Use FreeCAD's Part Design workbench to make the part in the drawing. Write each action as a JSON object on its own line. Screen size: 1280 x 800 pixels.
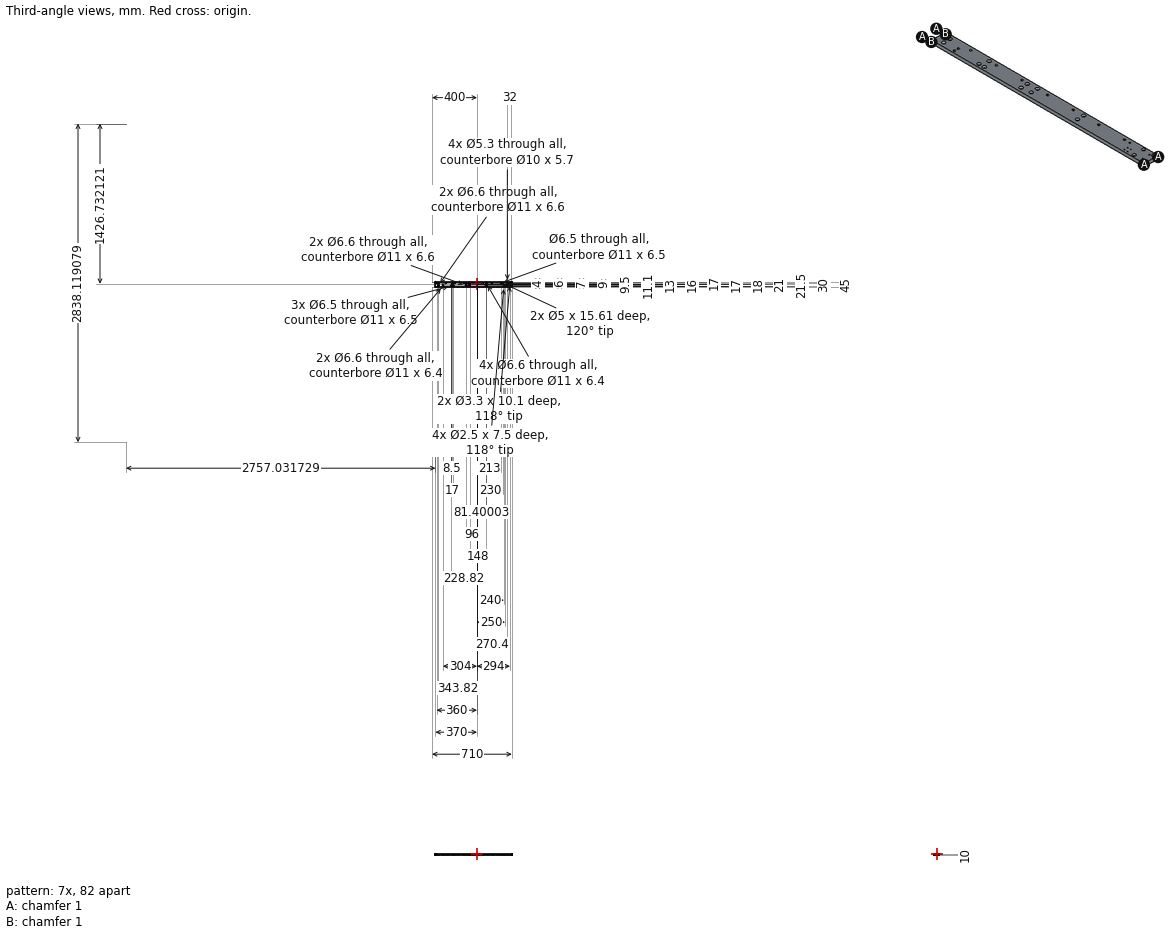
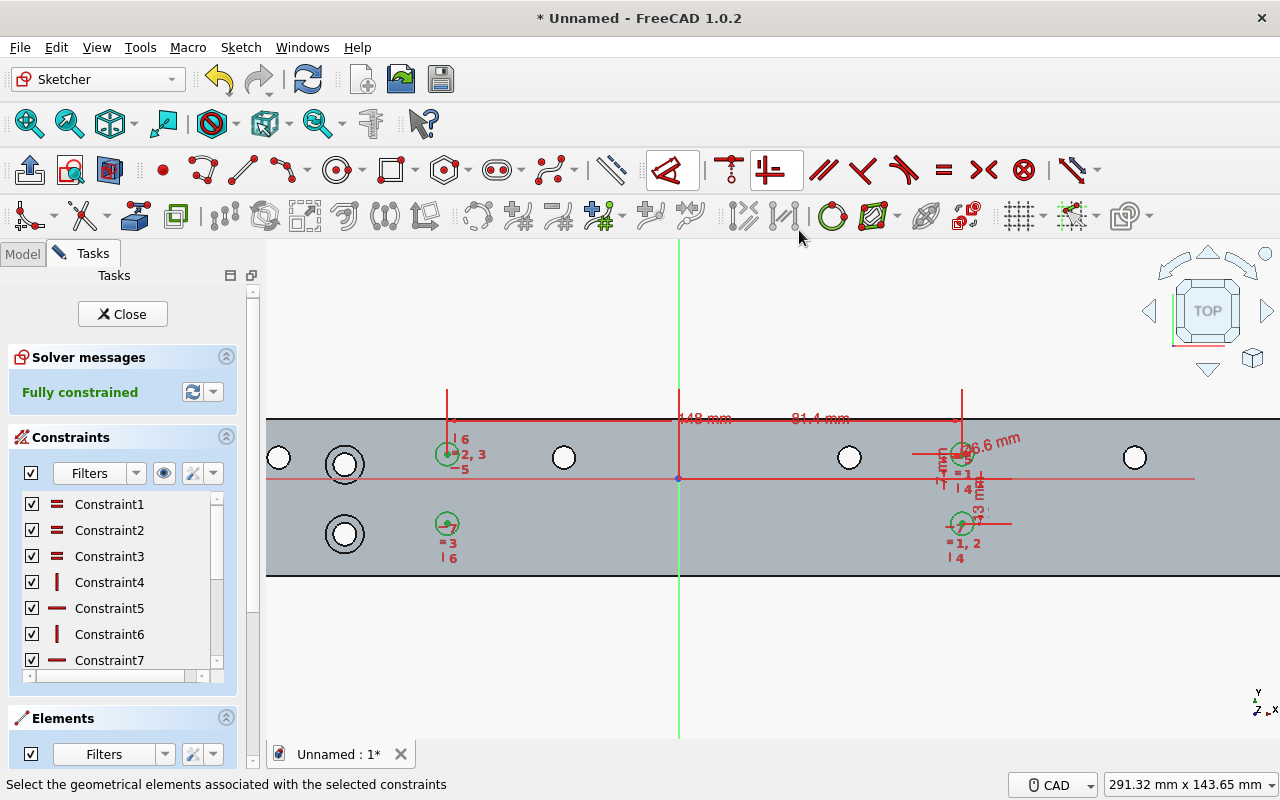
{"action": "left_click", "coordinate": [123, 314]}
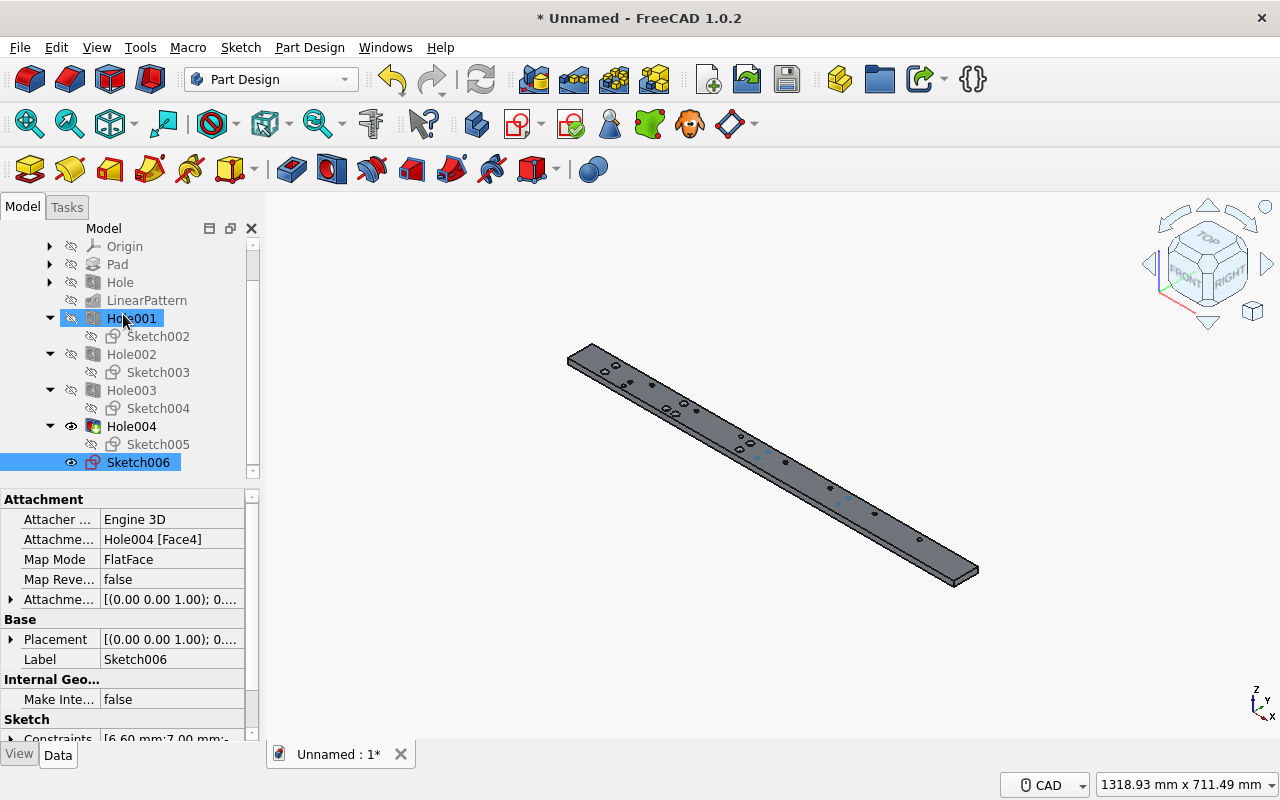
{"action": "left_click", "coordinate": [332, 170]}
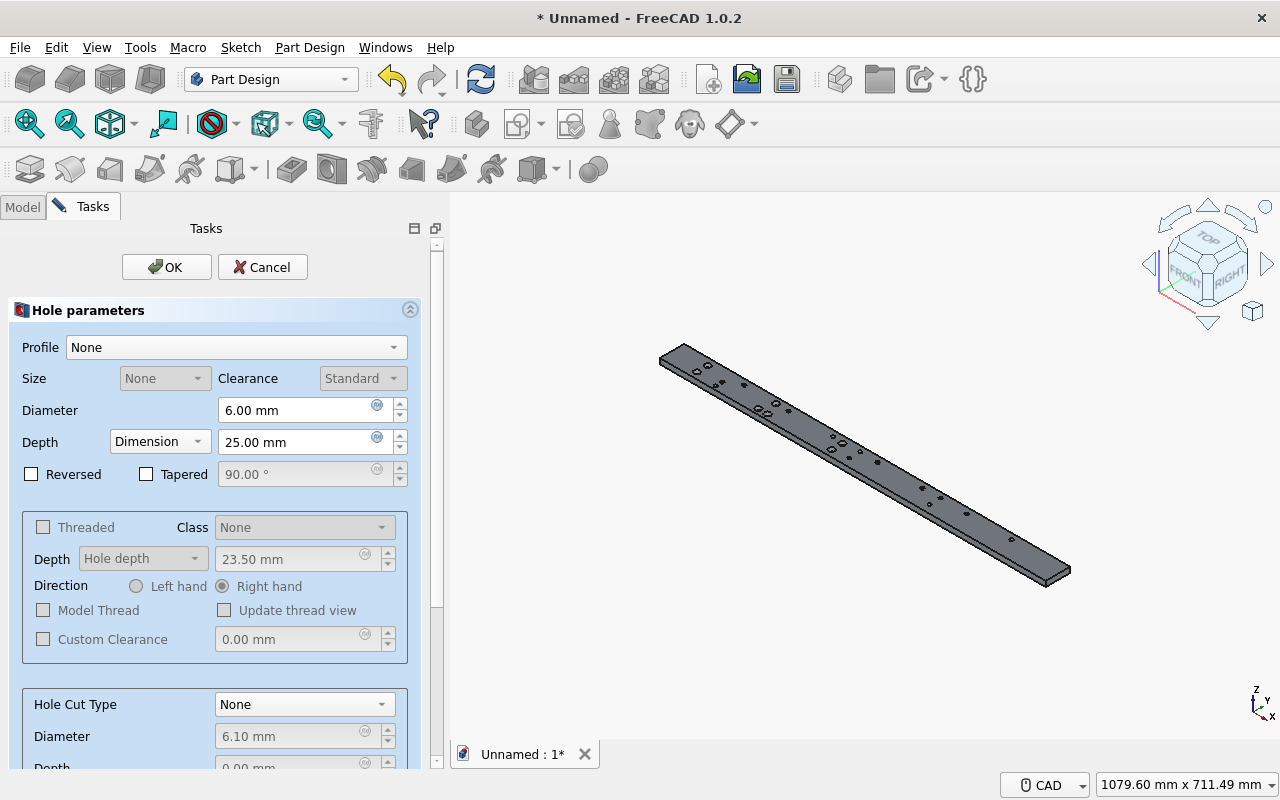
{"action": "triple_click", "coordinate": [305, 410]}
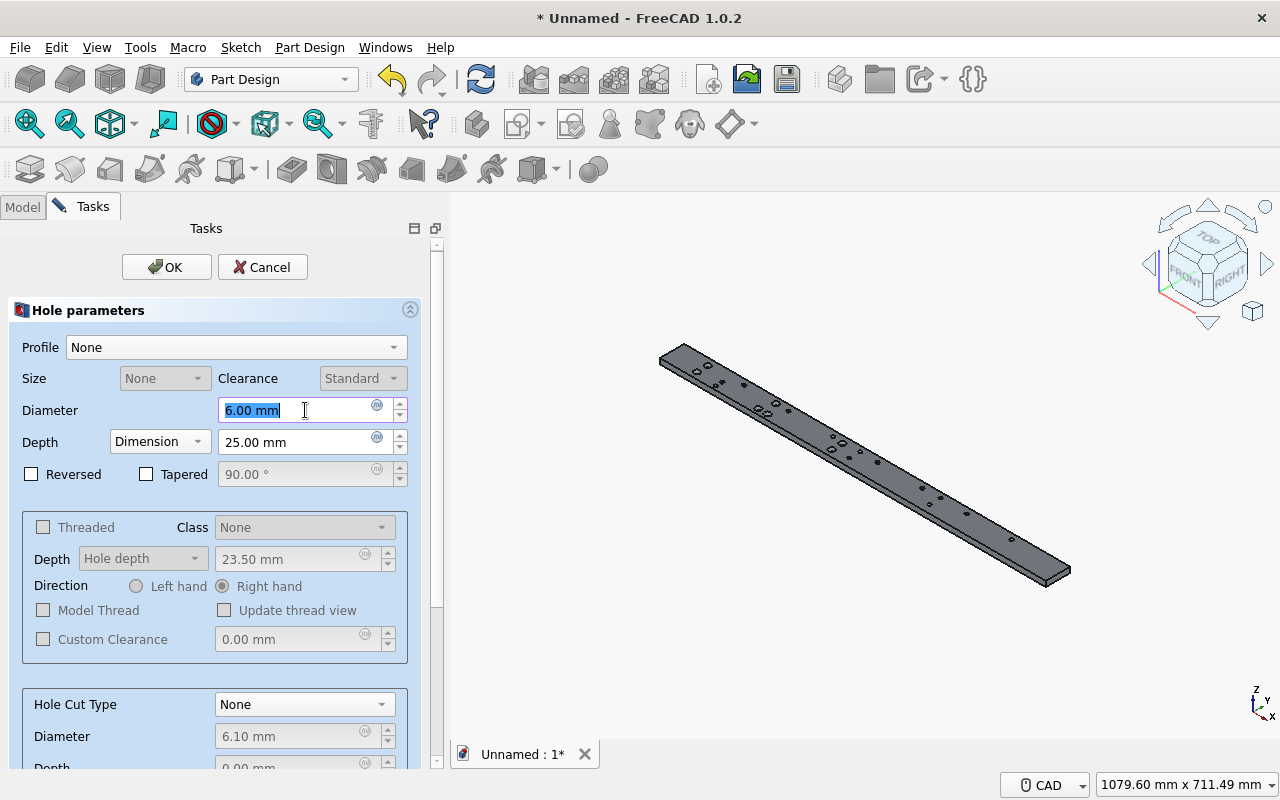
{"action": "type", "text": "6.6"}
{"action": "key", "text": "Tab"}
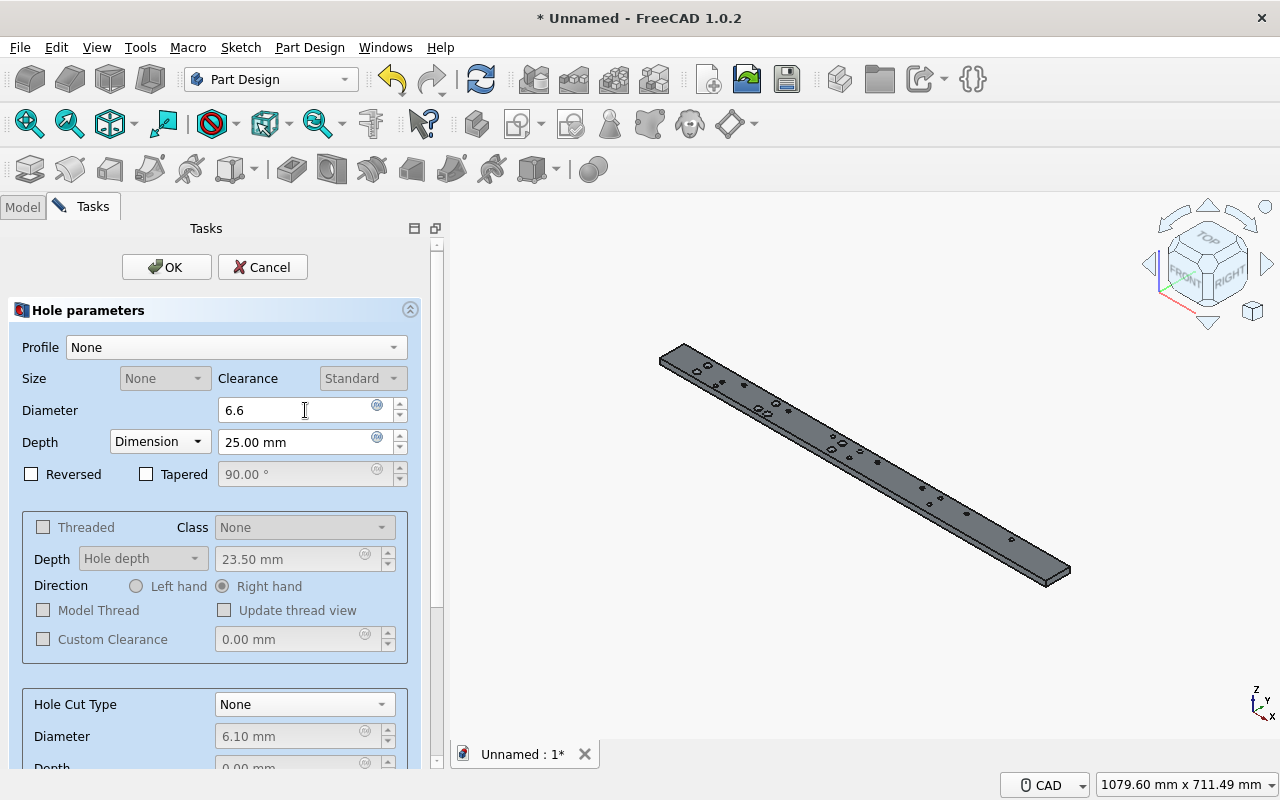
{"action": "left_click", "coordinate": [161, 442]}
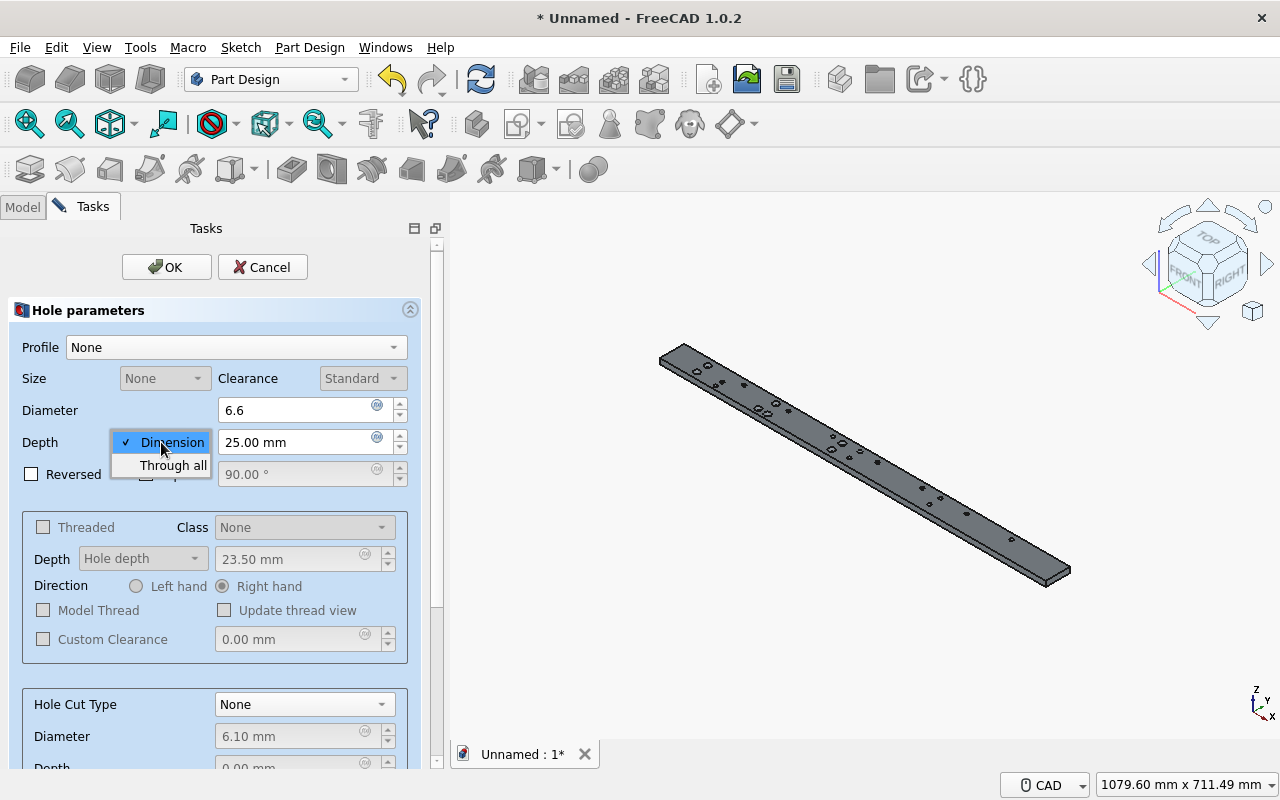
{"action": "left_click", "coordinate": [160, 466]}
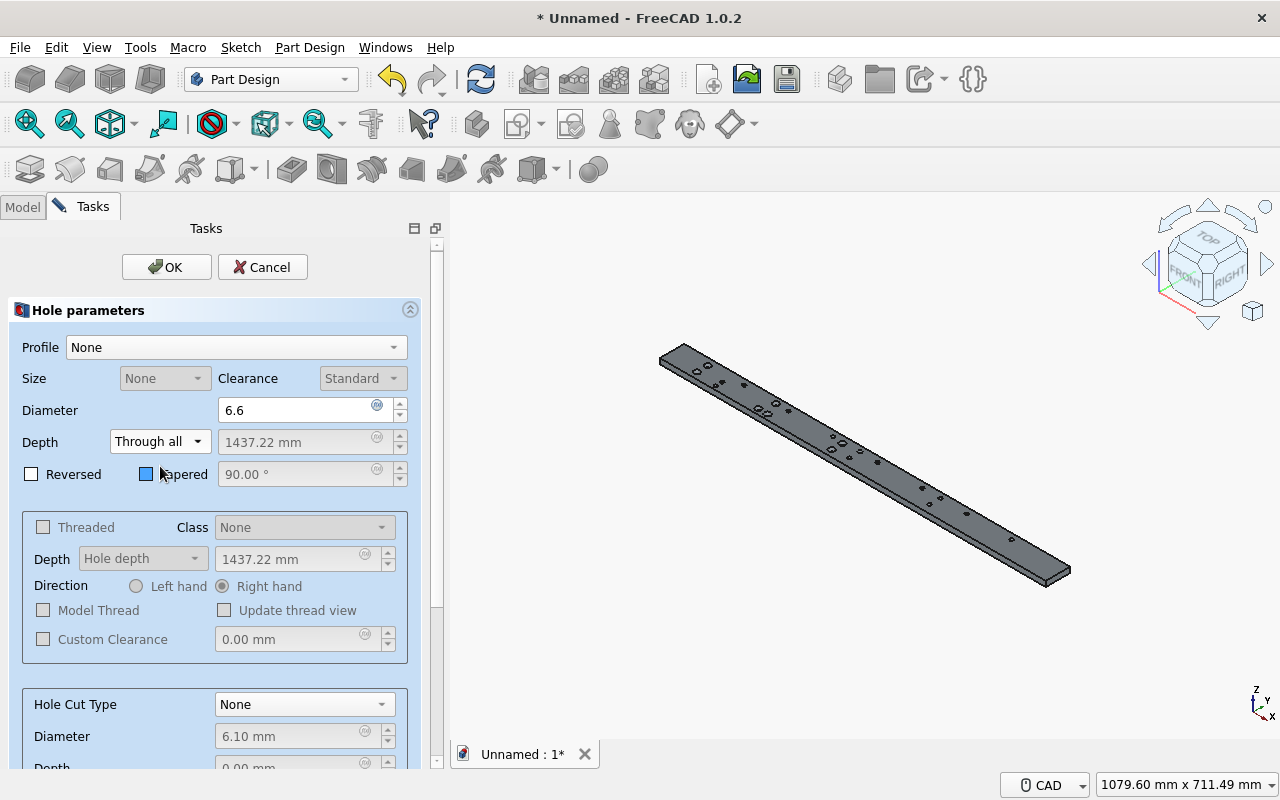
{"action": "left_click", "coordinate": [306, 704]}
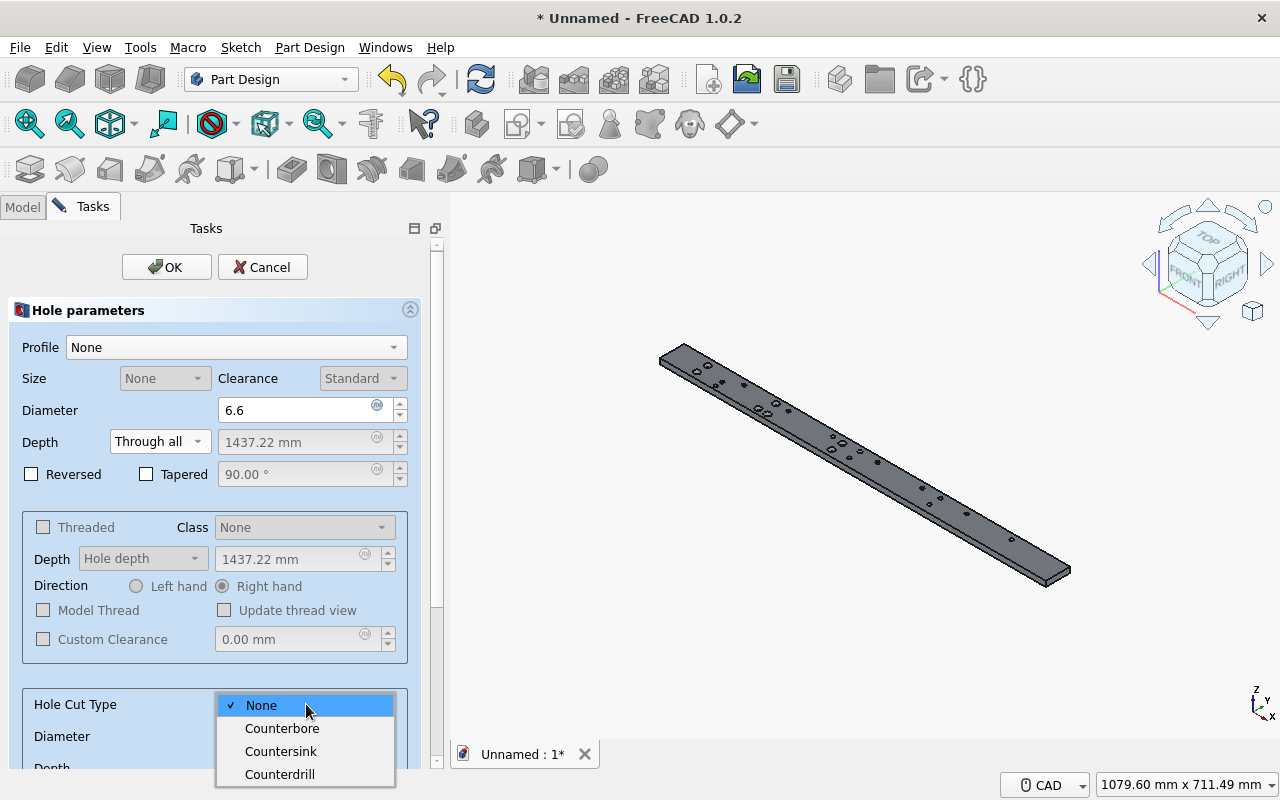
{"action": "left_click", "coordinate": [304, 728]}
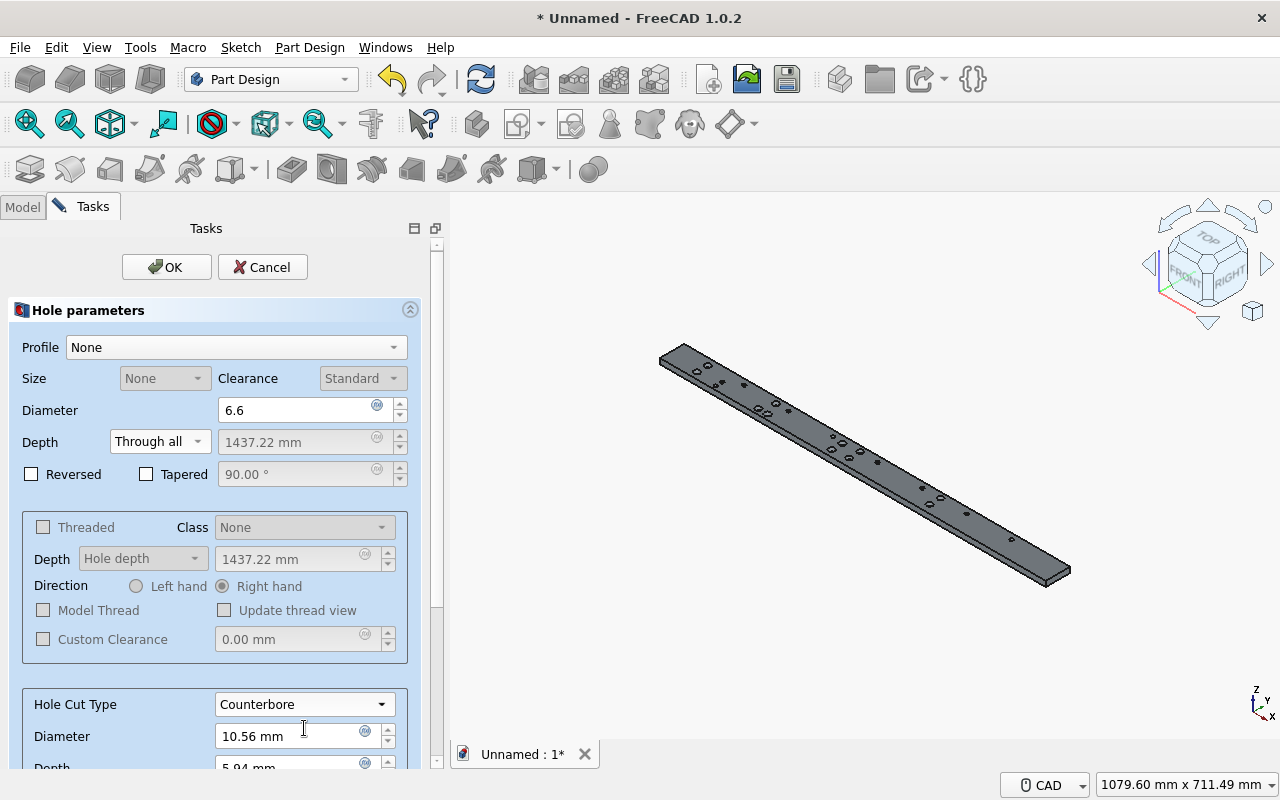
{"action": "triple_click", "coordinate": [298, 736]}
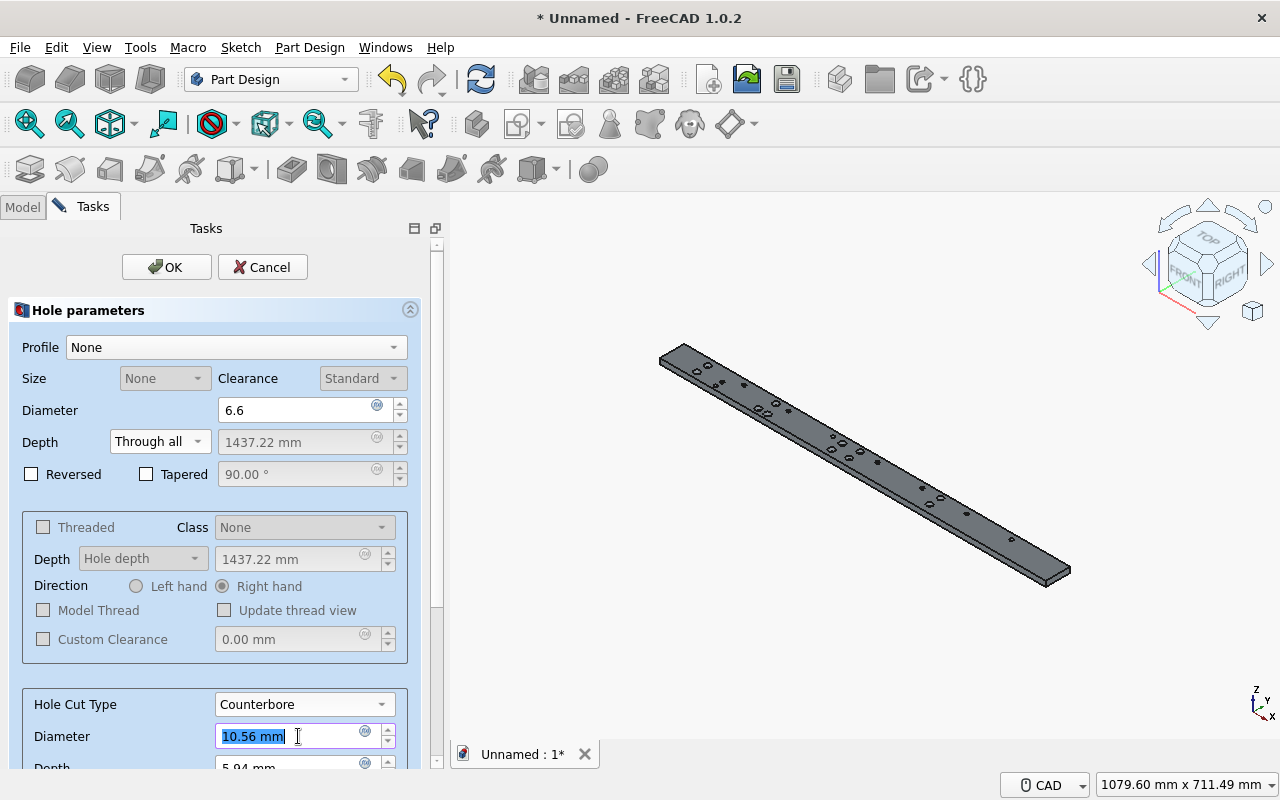
{"action": "type", "text": "11"}
{"action": "key", "text": "Tab"}